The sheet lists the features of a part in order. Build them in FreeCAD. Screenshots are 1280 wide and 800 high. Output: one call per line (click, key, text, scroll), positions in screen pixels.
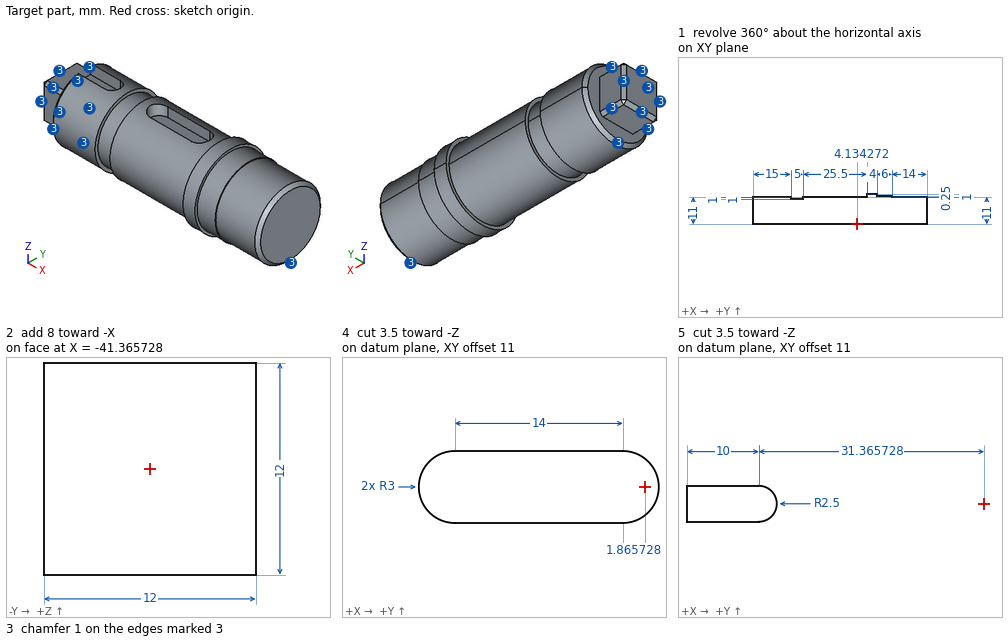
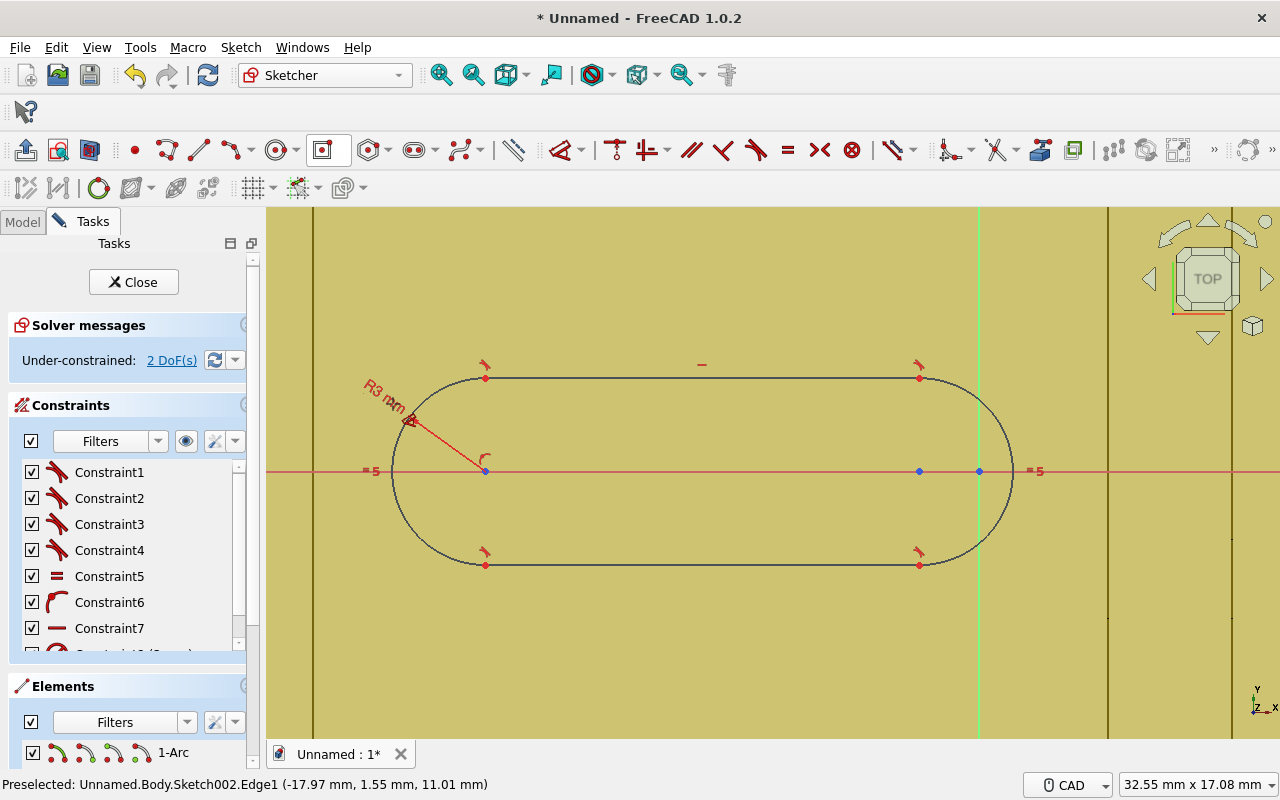
click(616, 378)
click(703, 344)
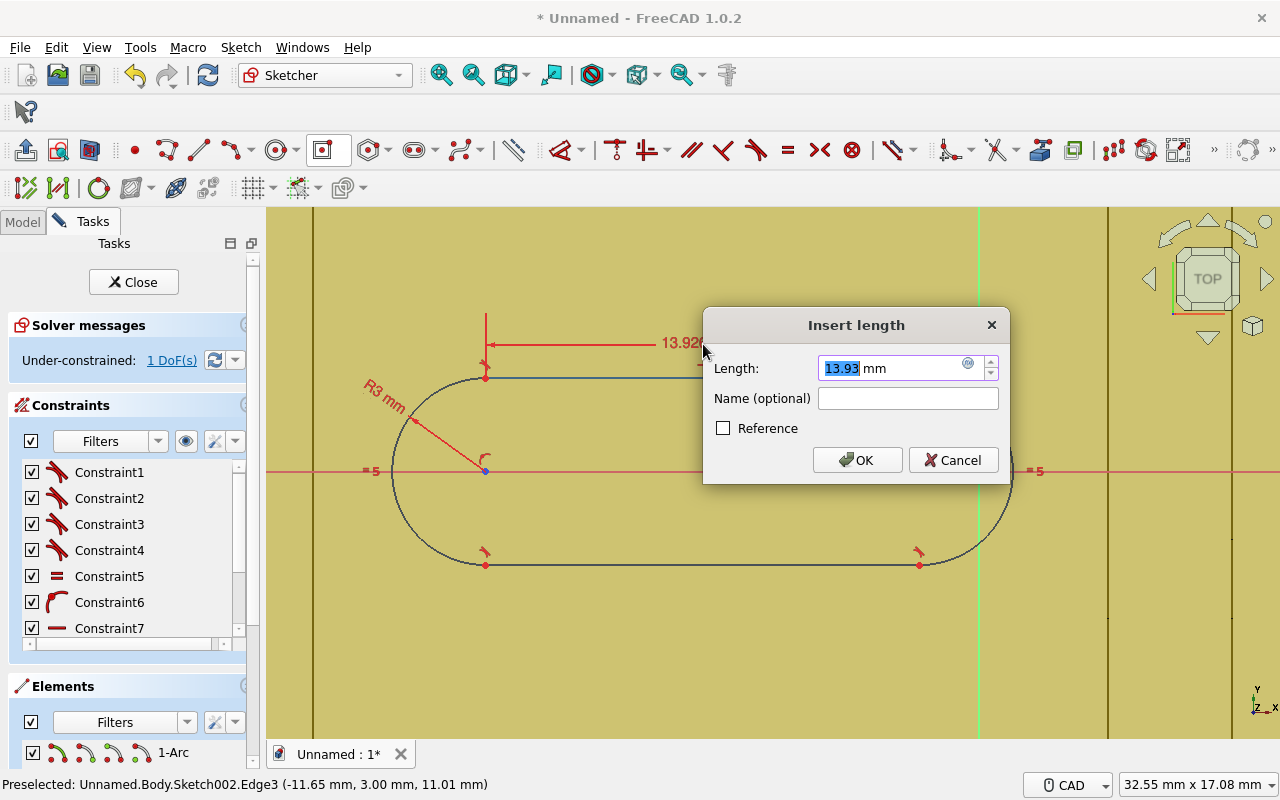
text(14)
key(Return)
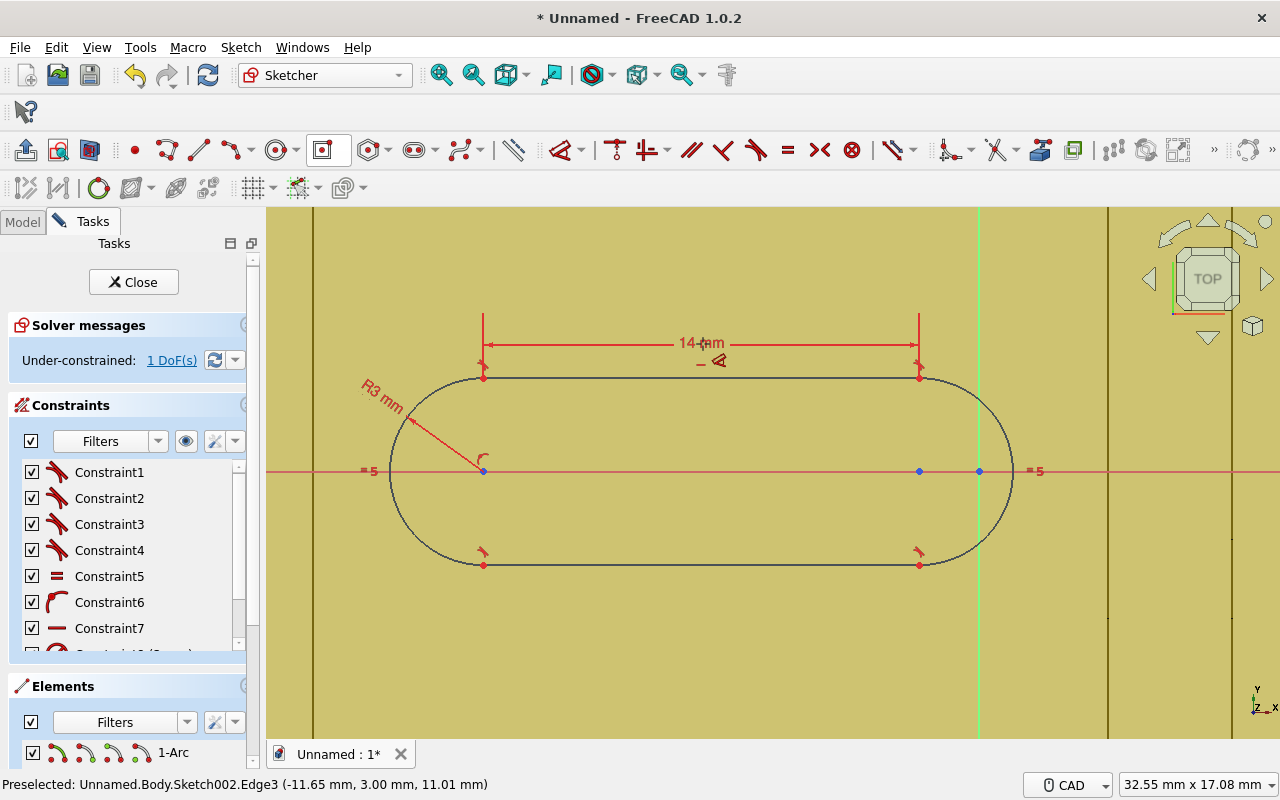
click(919, 565)
click(949, 599)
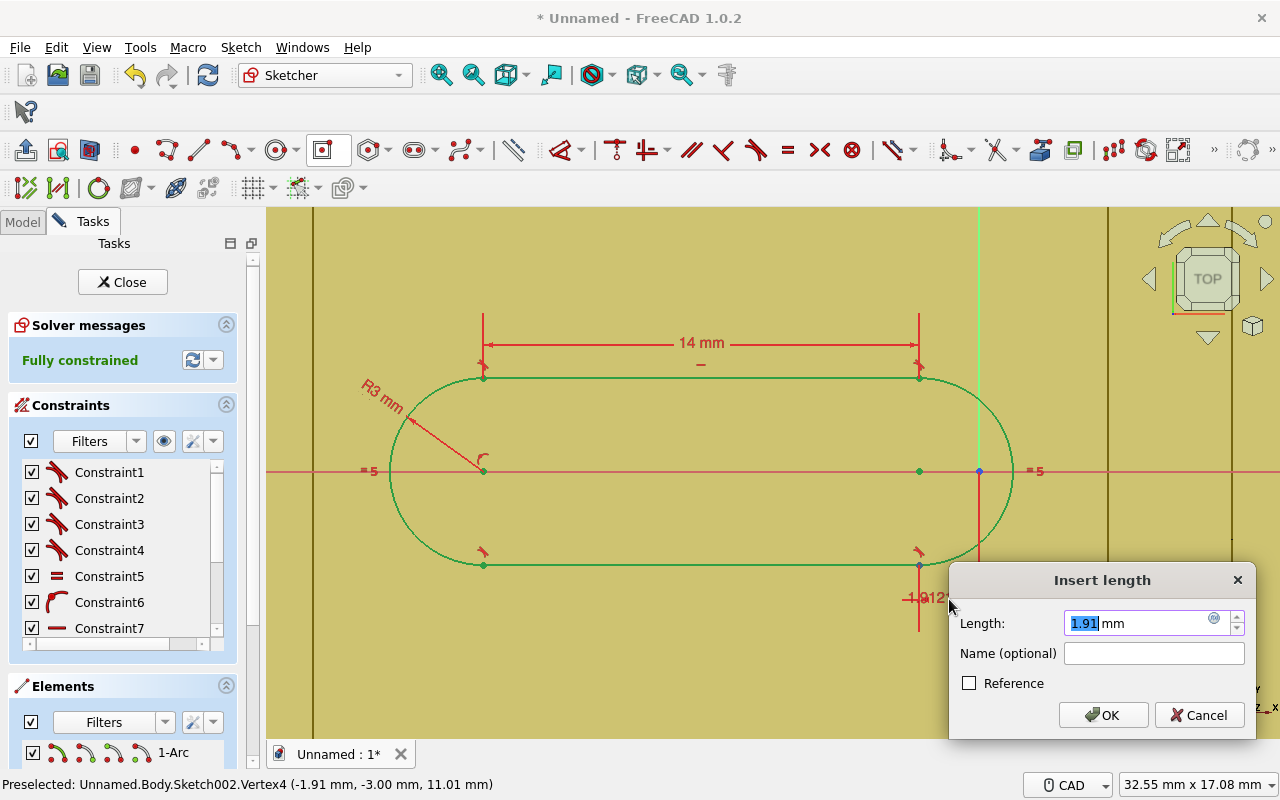
text(1.865728)
key(Return)
key(Escape)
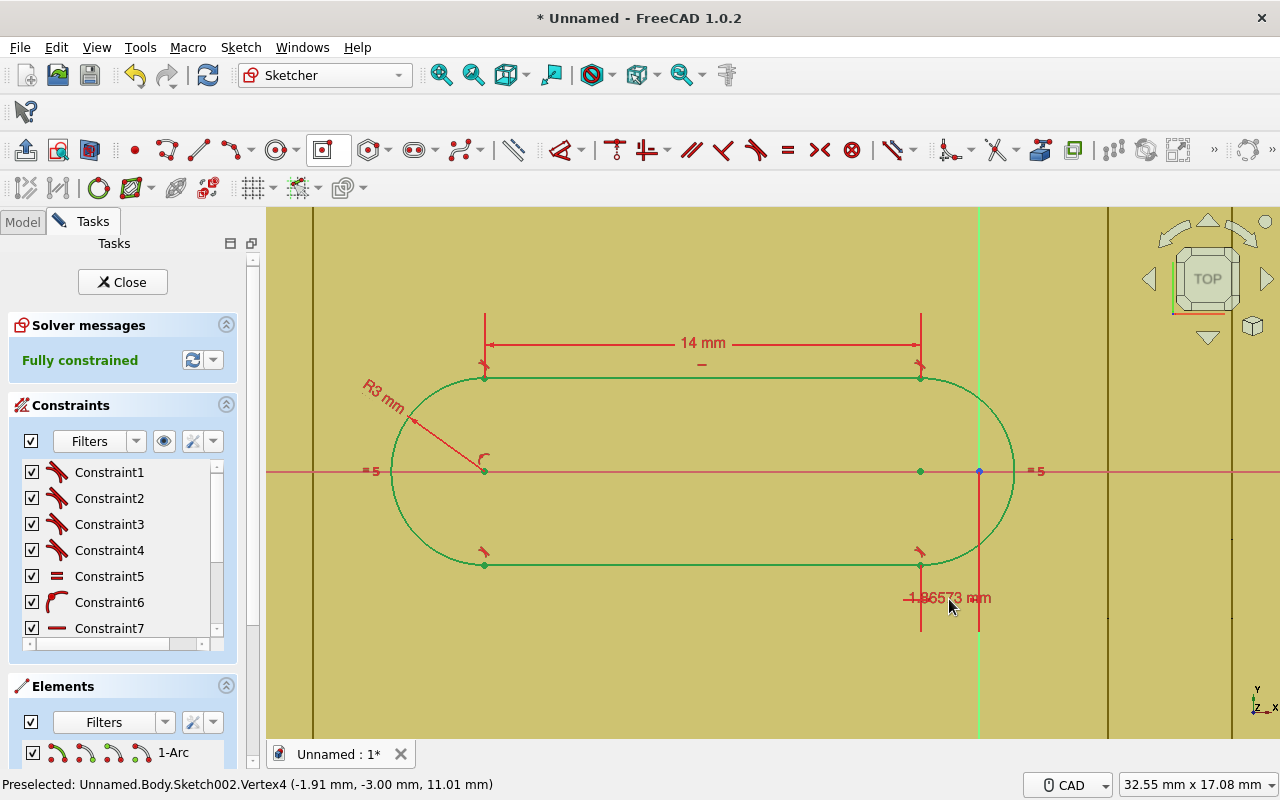
click(123, 282)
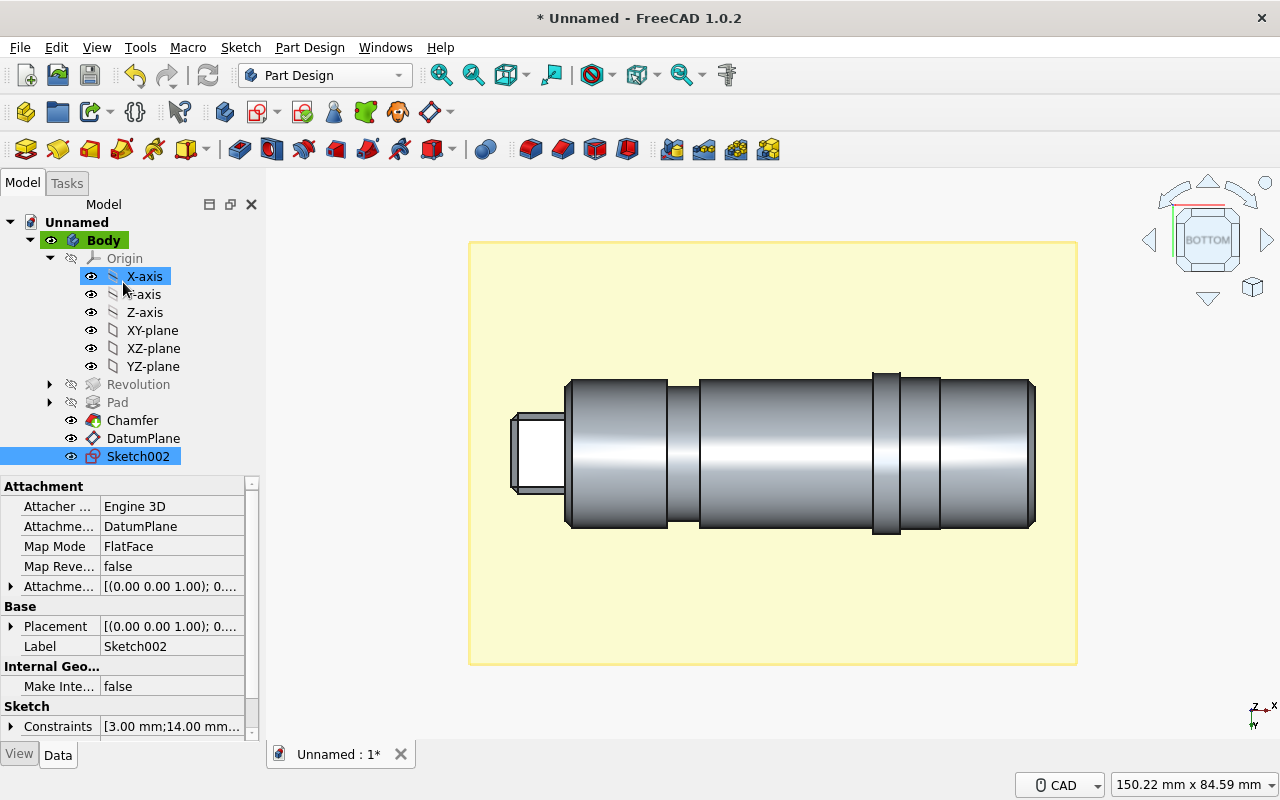
click(240, 150)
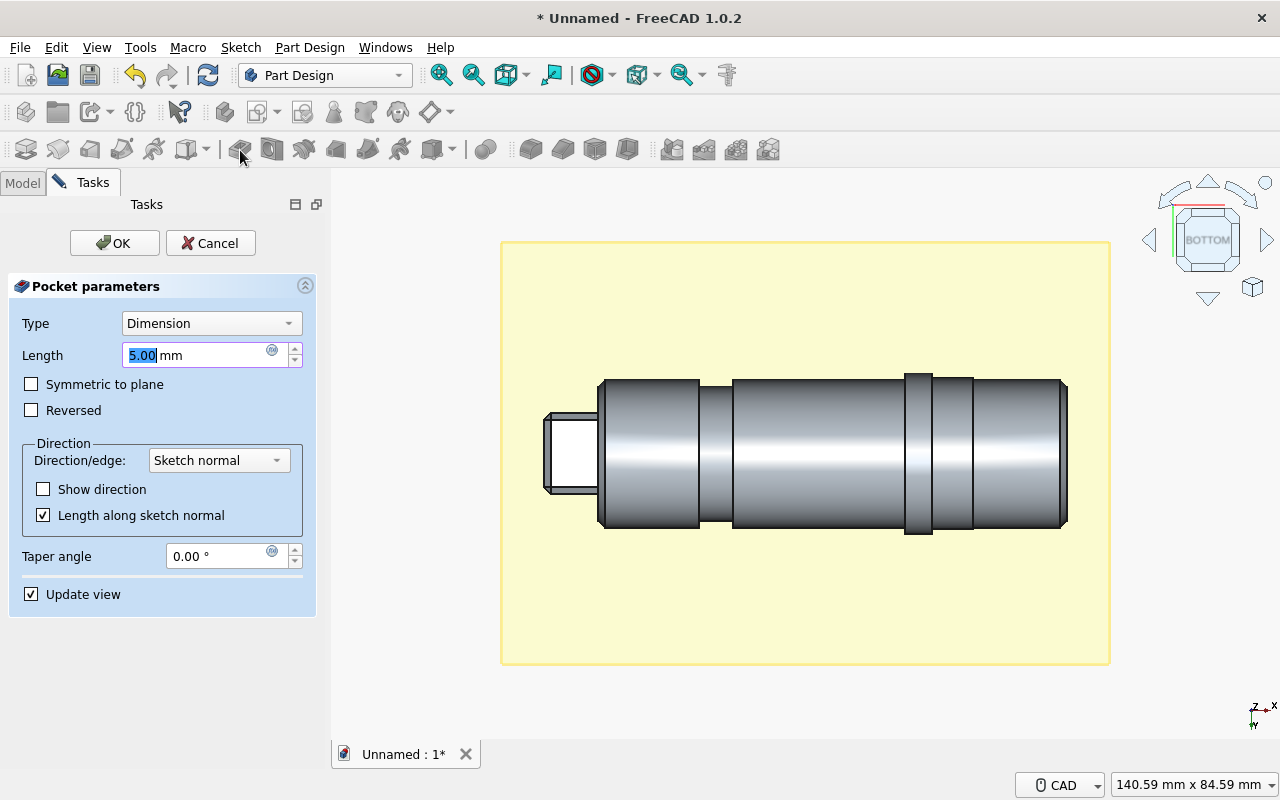
text(3.5)
key(Tab)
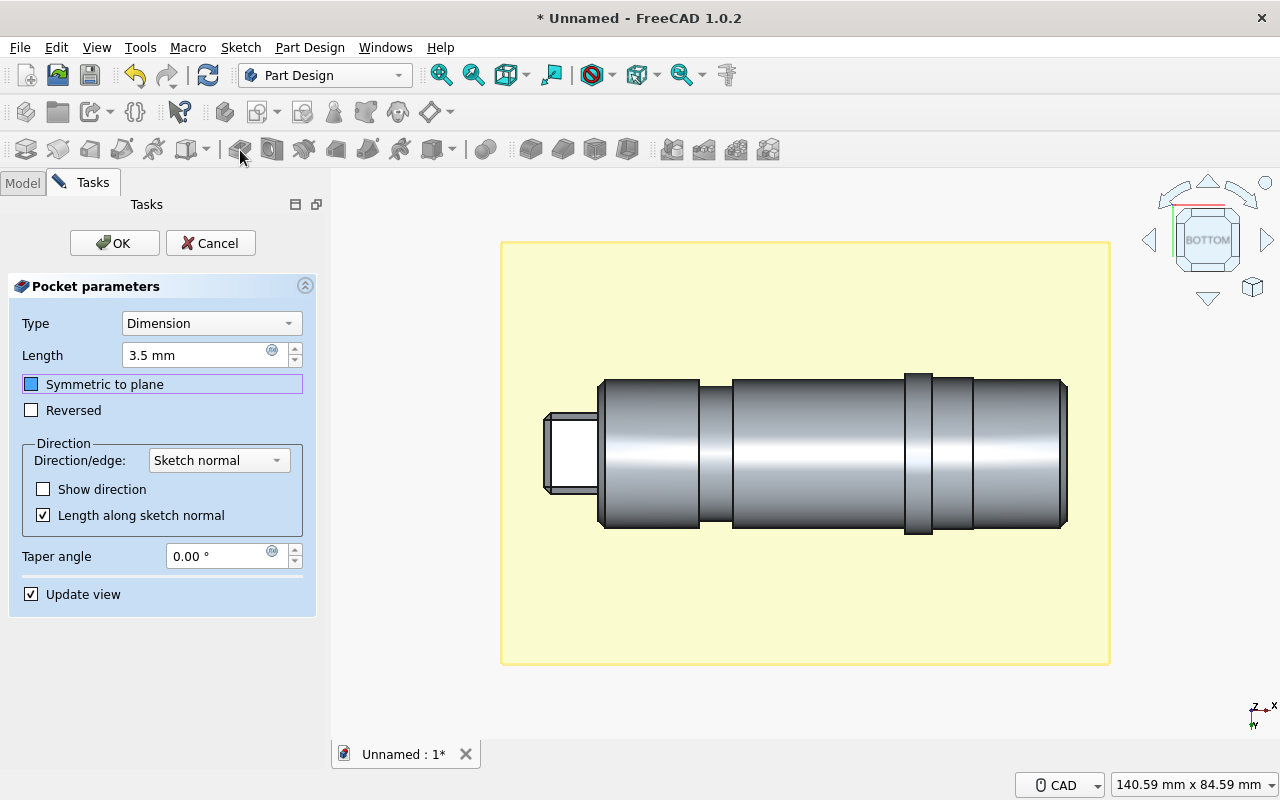
click(115, 243)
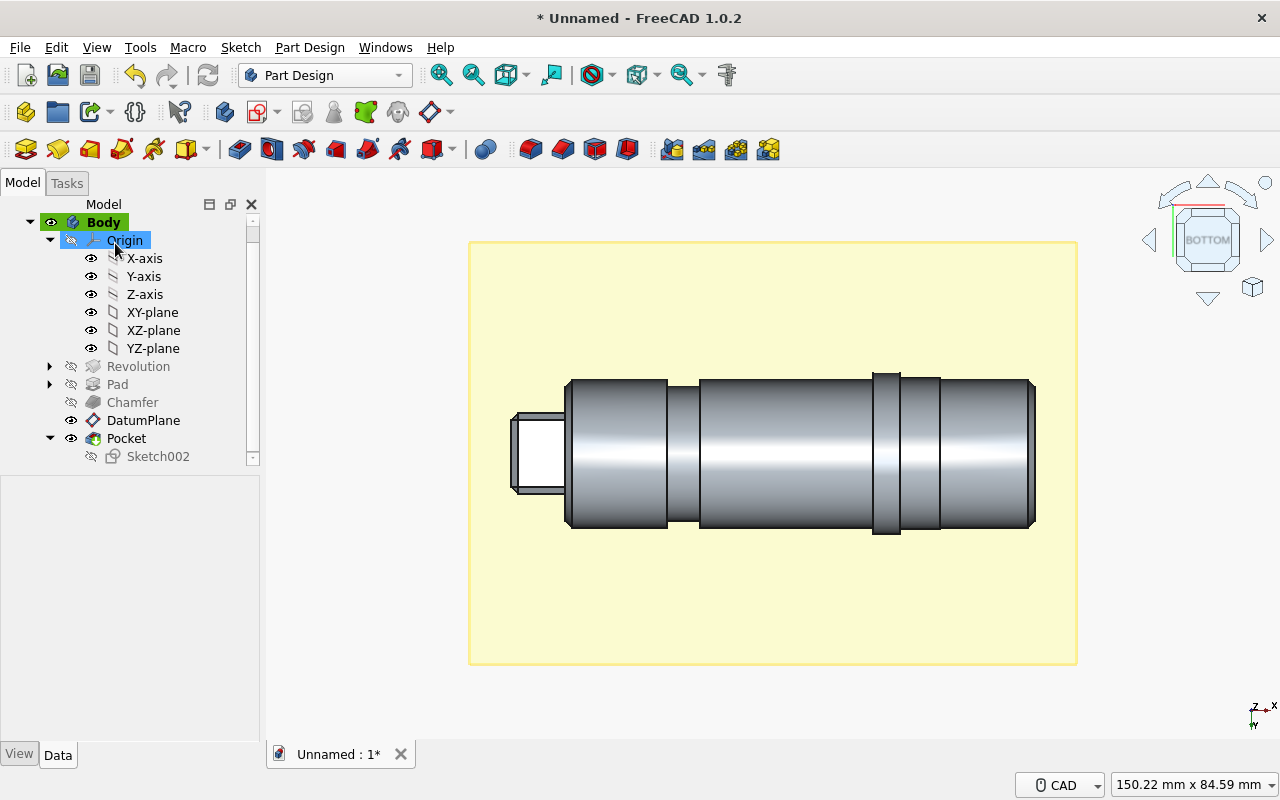
click(116, 420)
key(space)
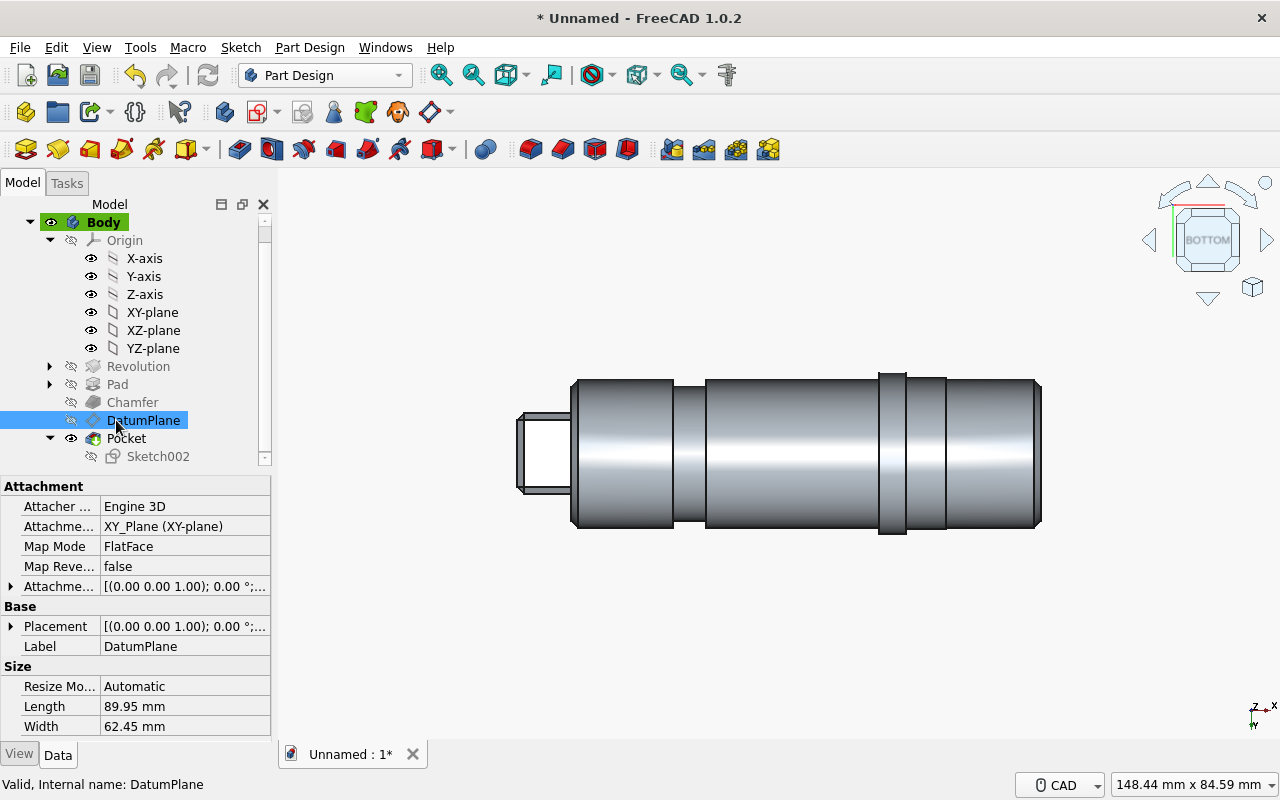
click(136, 312)